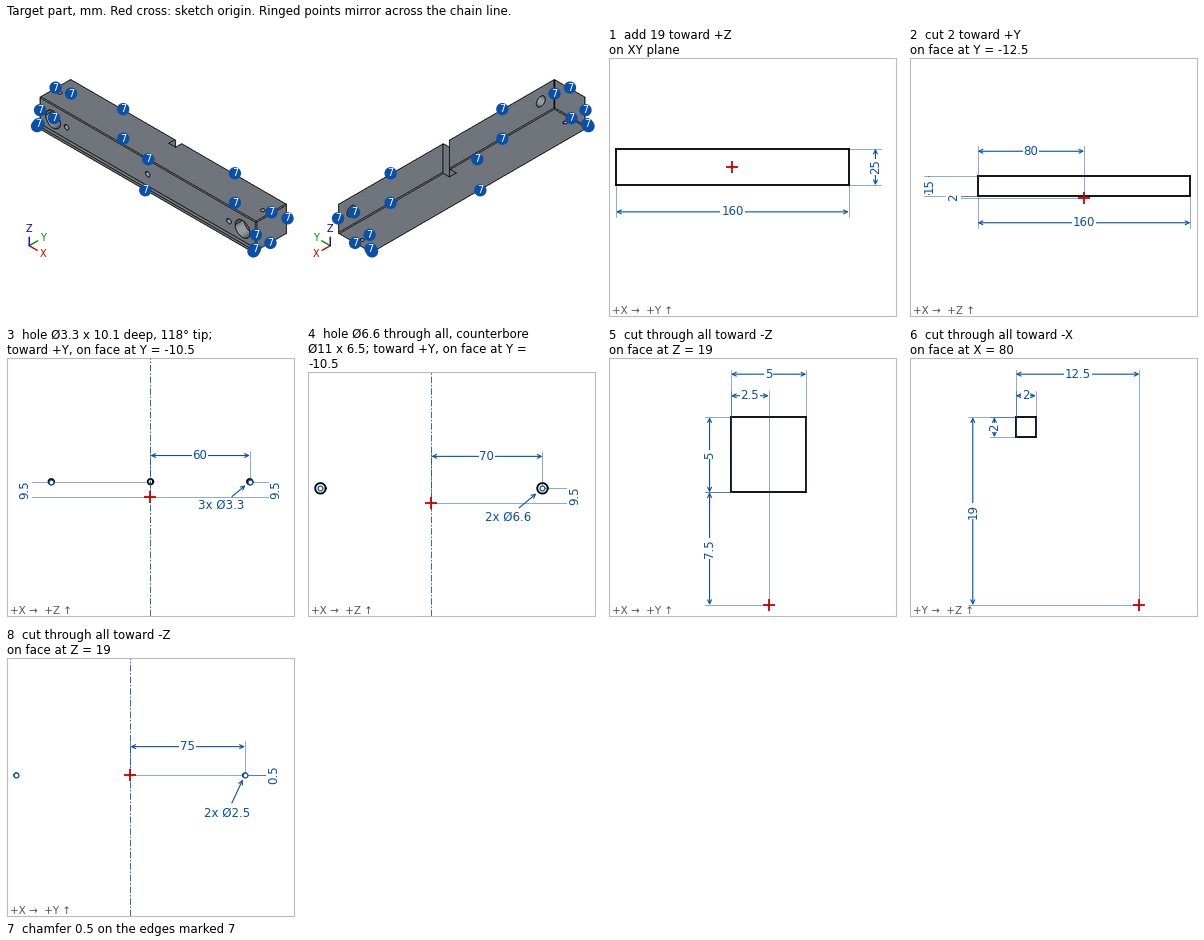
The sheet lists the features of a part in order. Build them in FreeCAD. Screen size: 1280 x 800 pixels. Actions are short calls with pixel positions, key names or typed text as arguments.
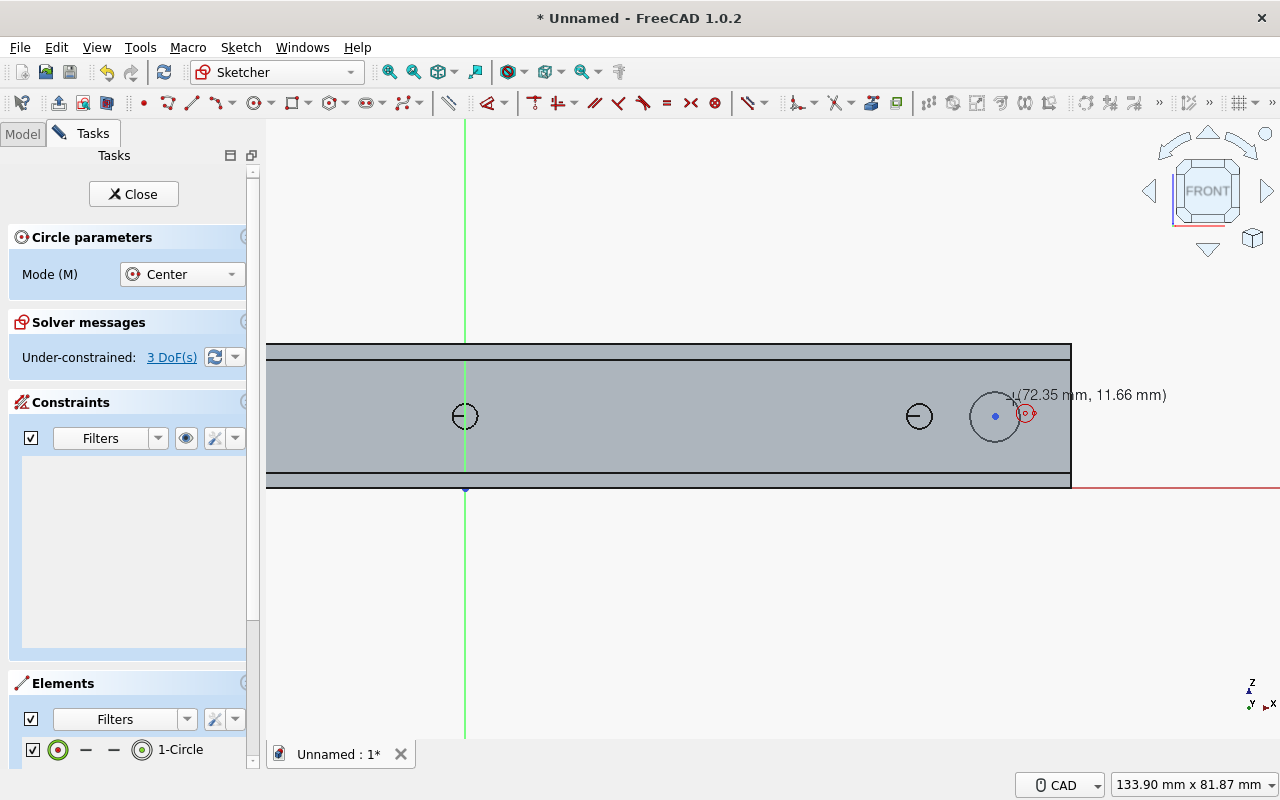
scroll(996, 416, down, 3)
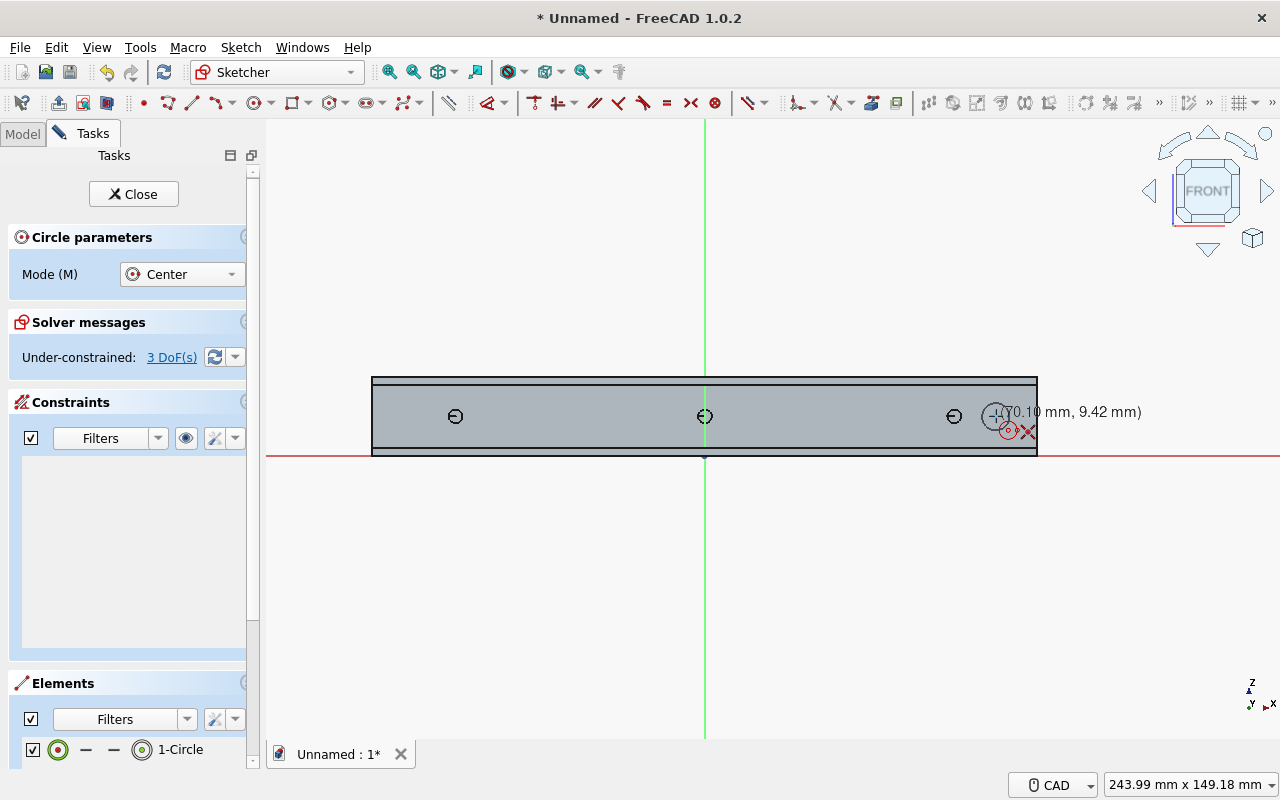
scroll(414, 416, up, 3)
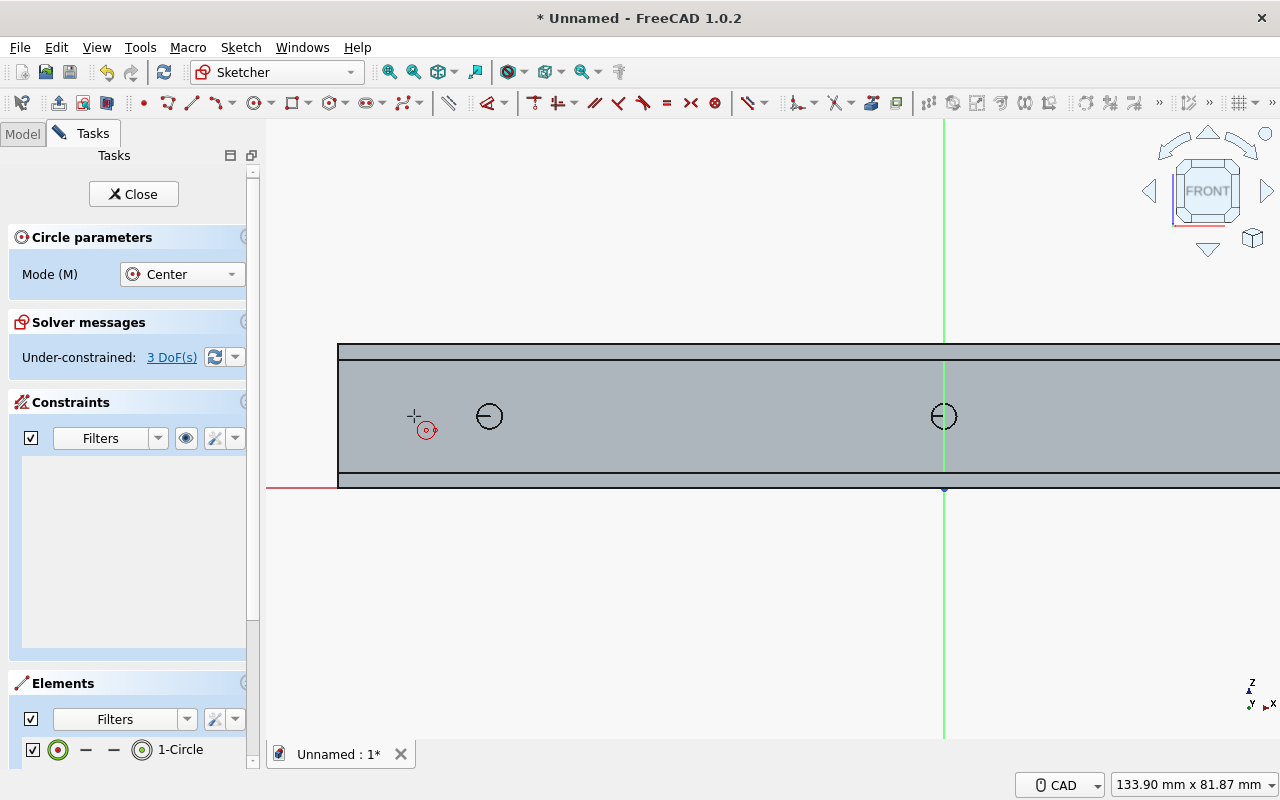
click(414, 416)
click(432, 399)
key(Escape)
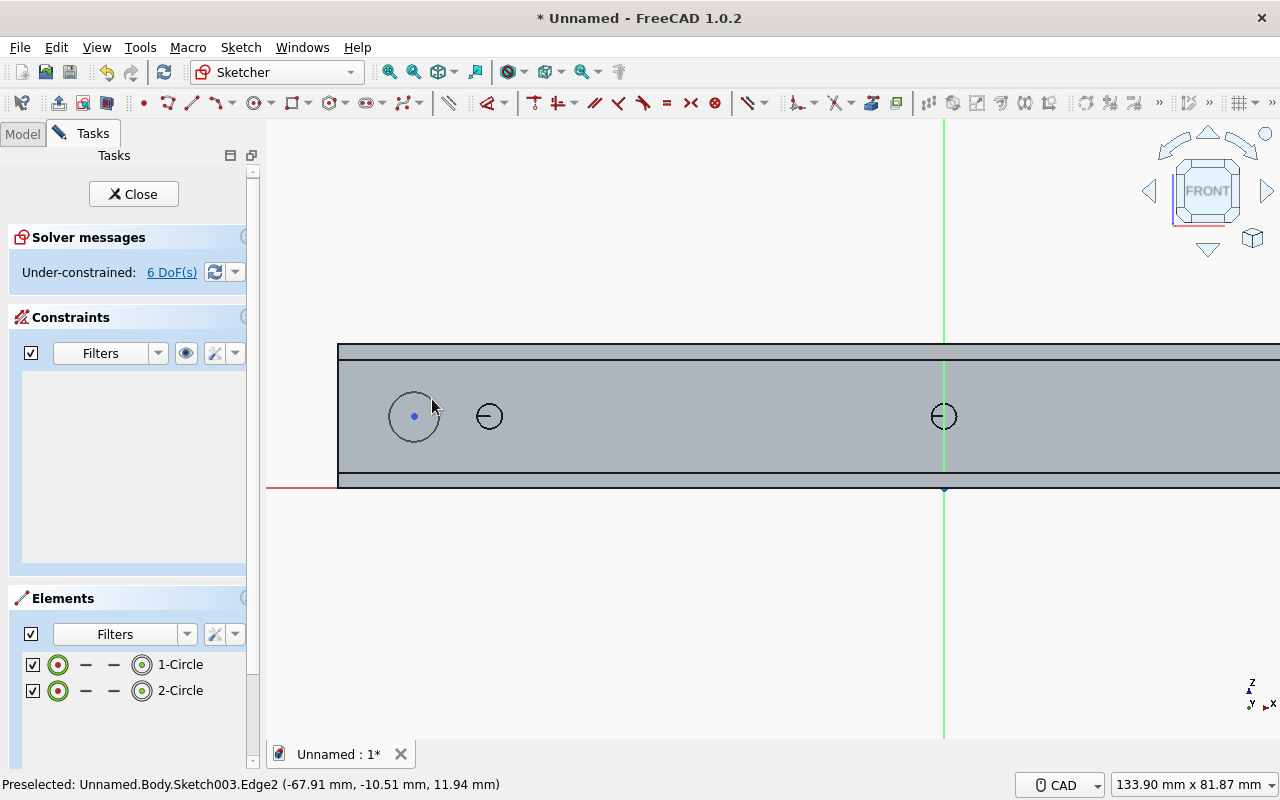
scroll(413, 416, down, 3)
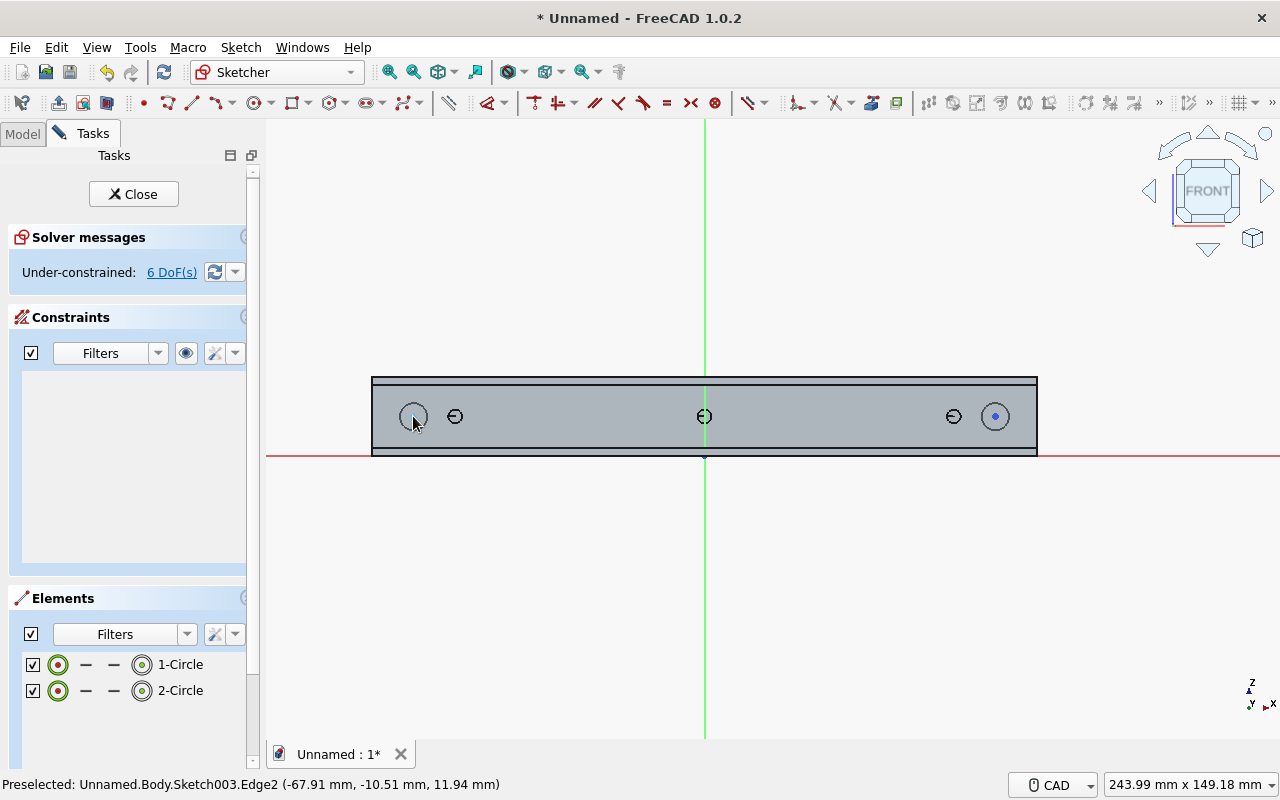
click(1005, 407)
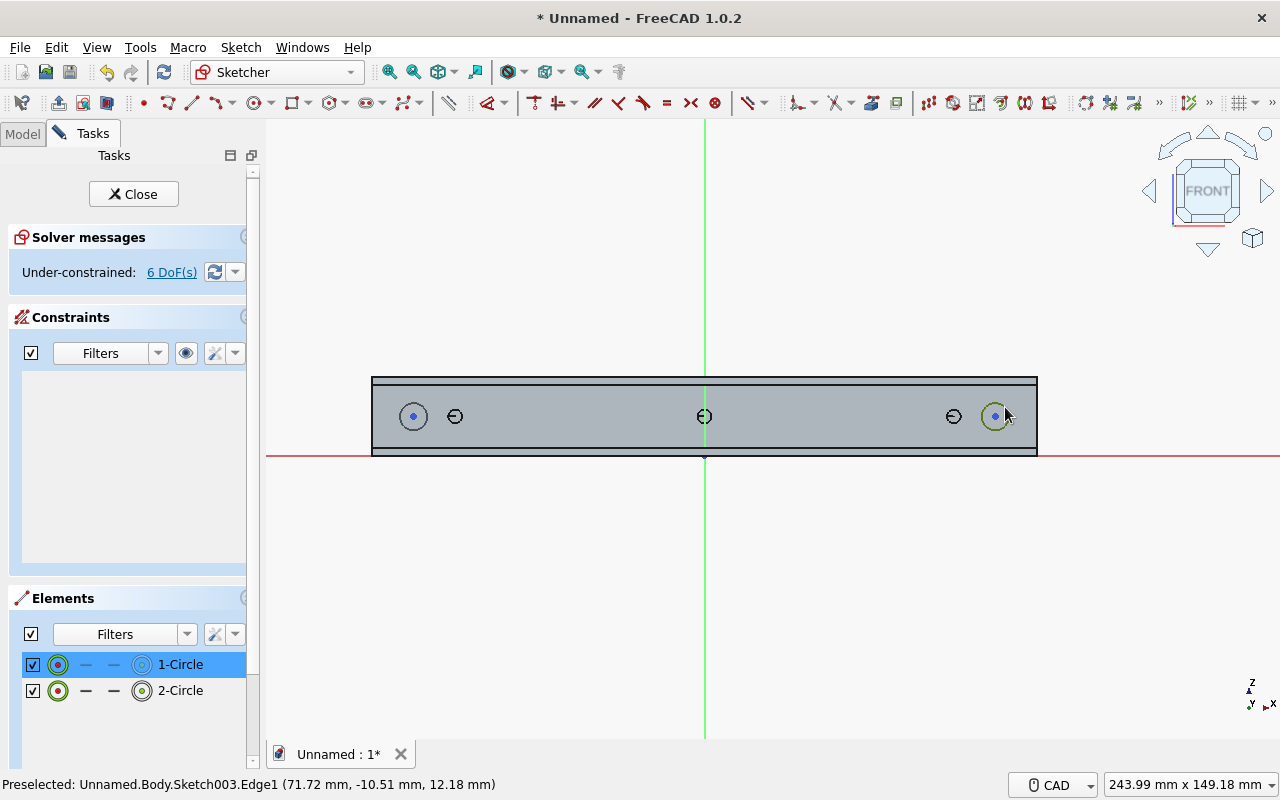
click(423, 407)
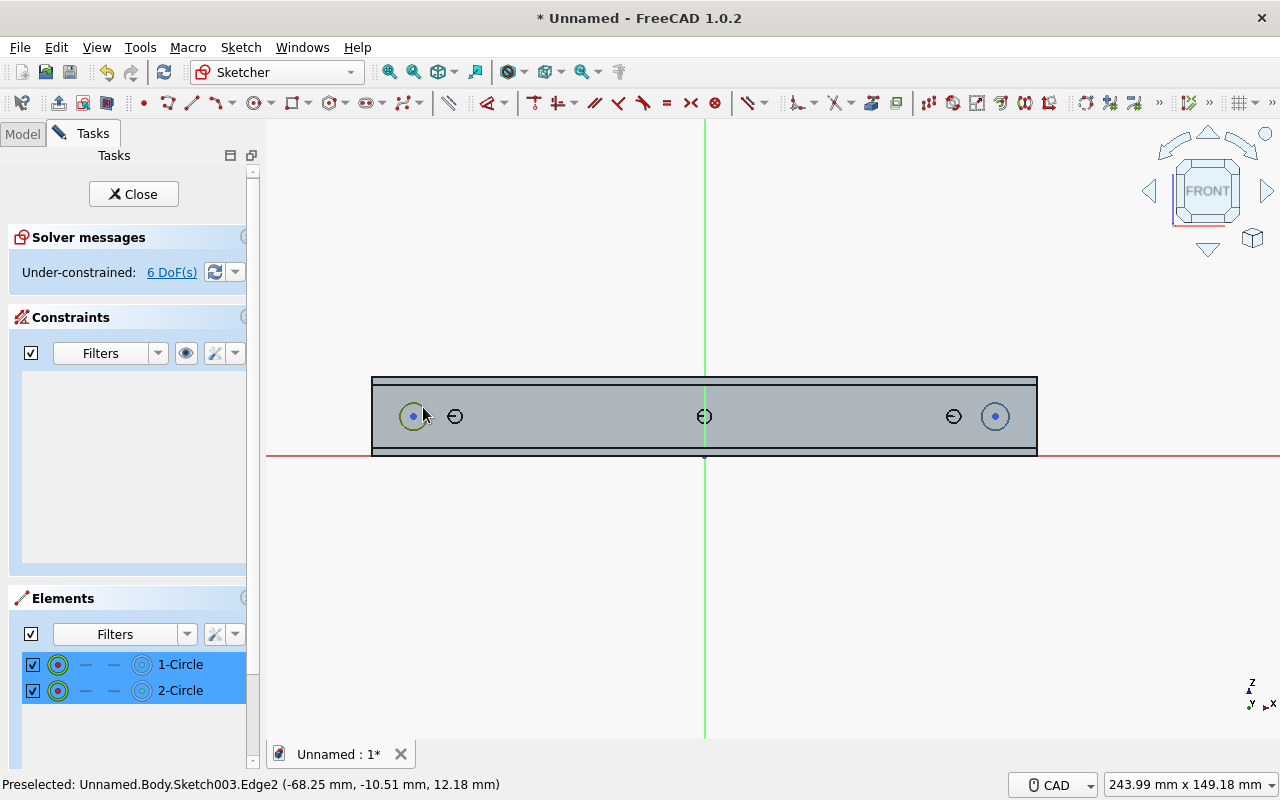
click(668, 104)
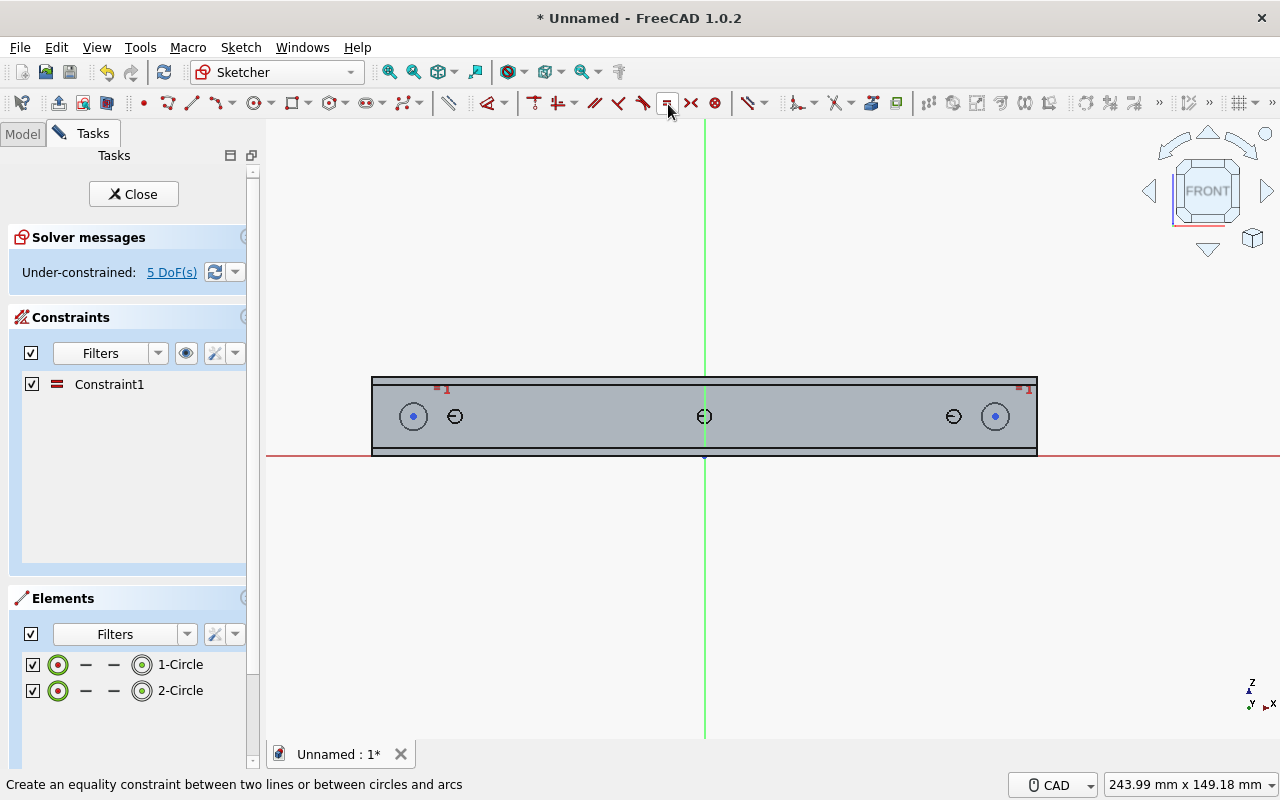
click(995, 417)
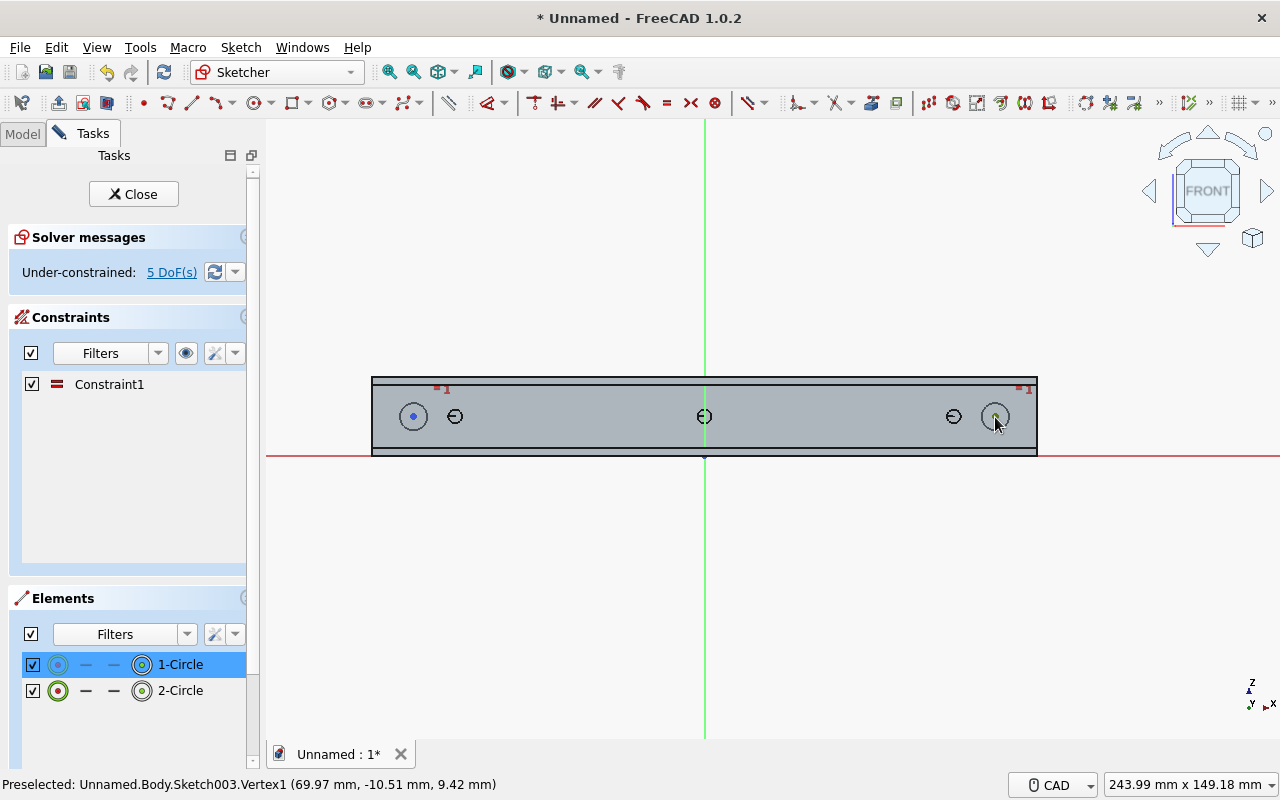
click(414, 417)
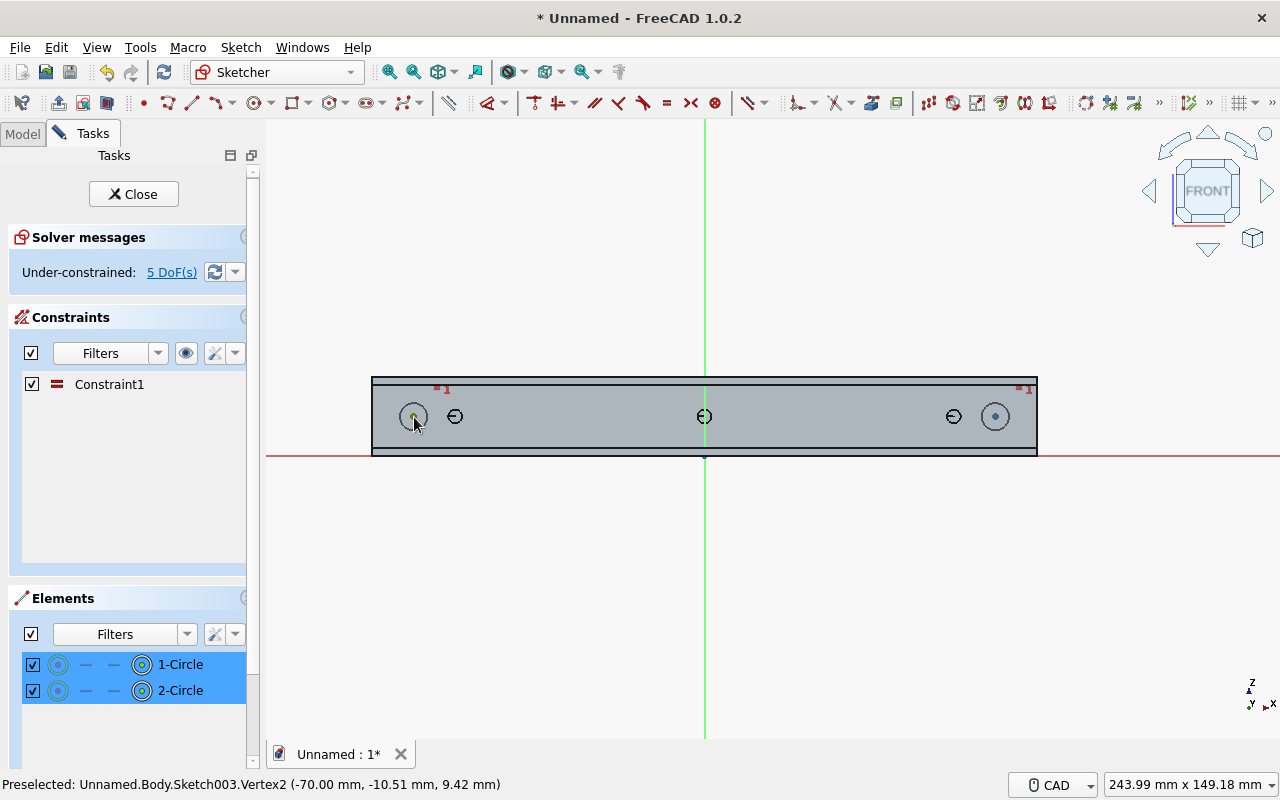
click(705, 671)